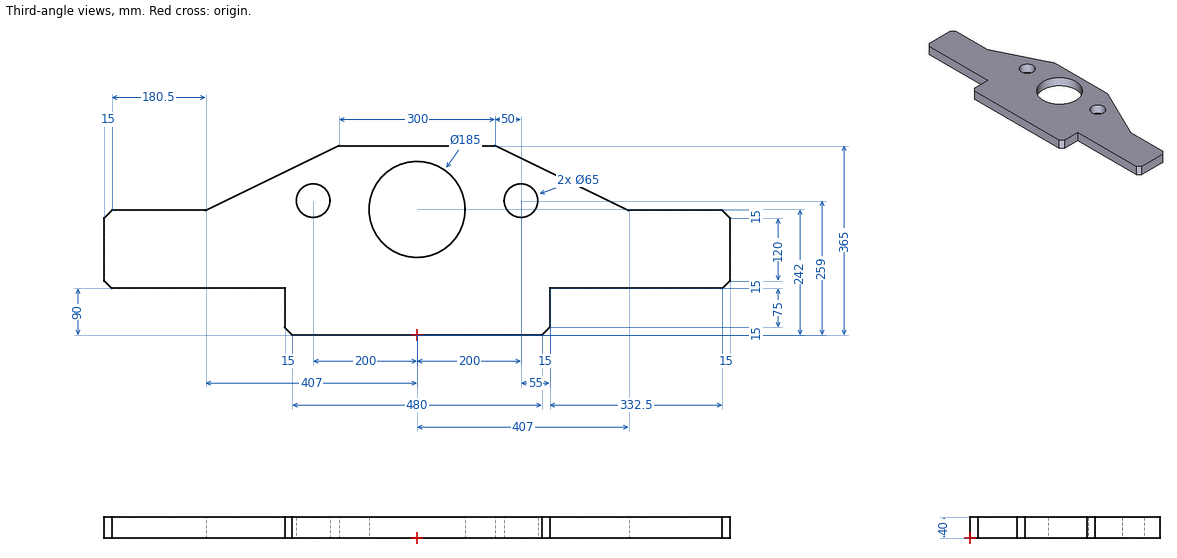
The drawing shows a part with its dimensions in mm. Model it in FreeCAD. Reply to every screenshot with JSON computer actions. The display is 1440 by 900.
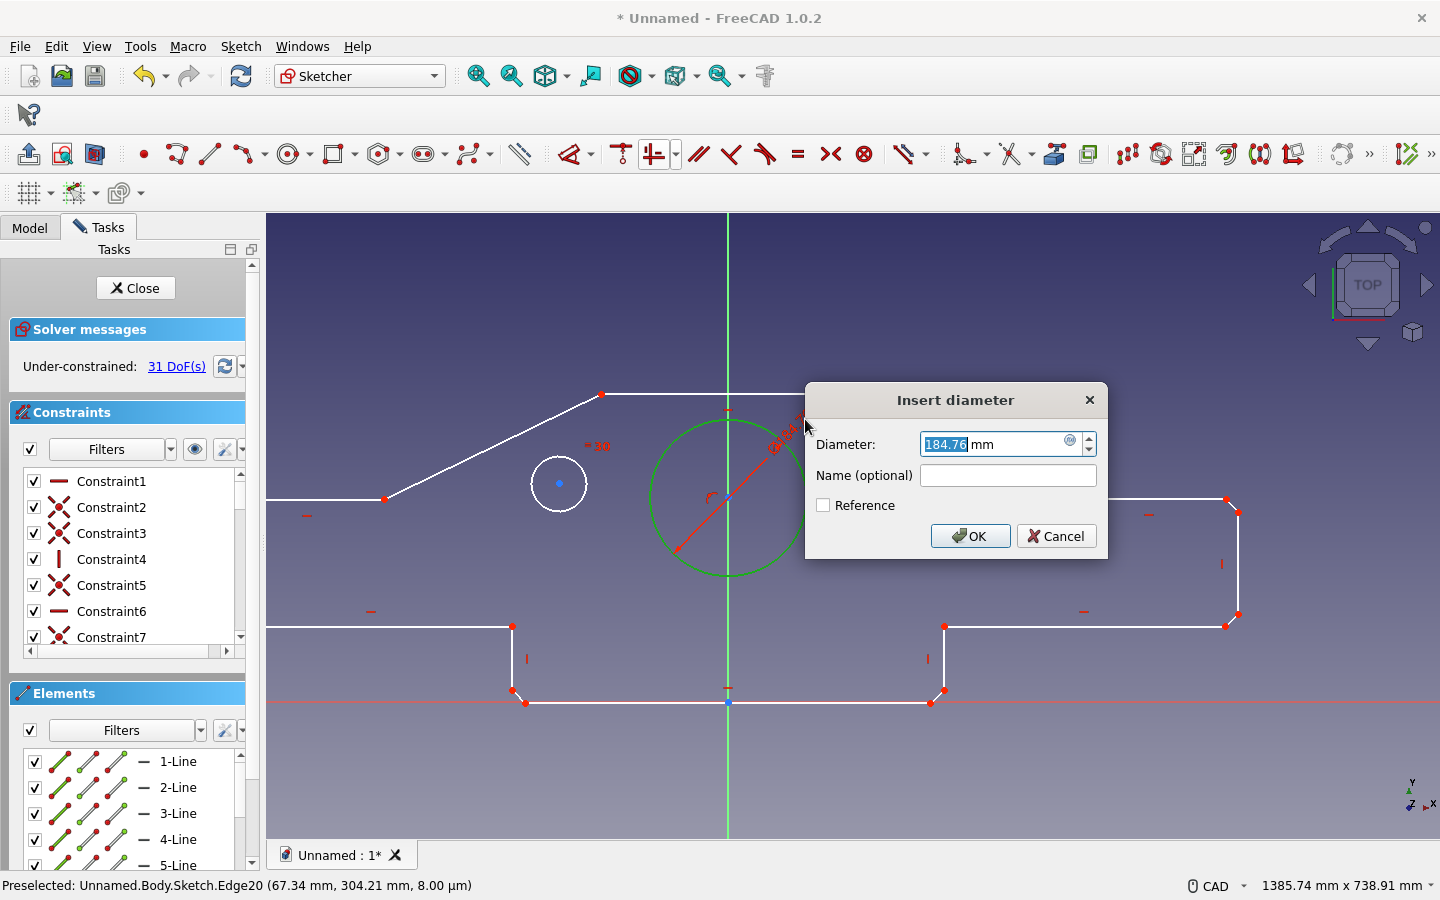
{"action": "type", "text": "185"}
{"action": "key", "text": "Return"}
{"action": "key", "text": "Escape"}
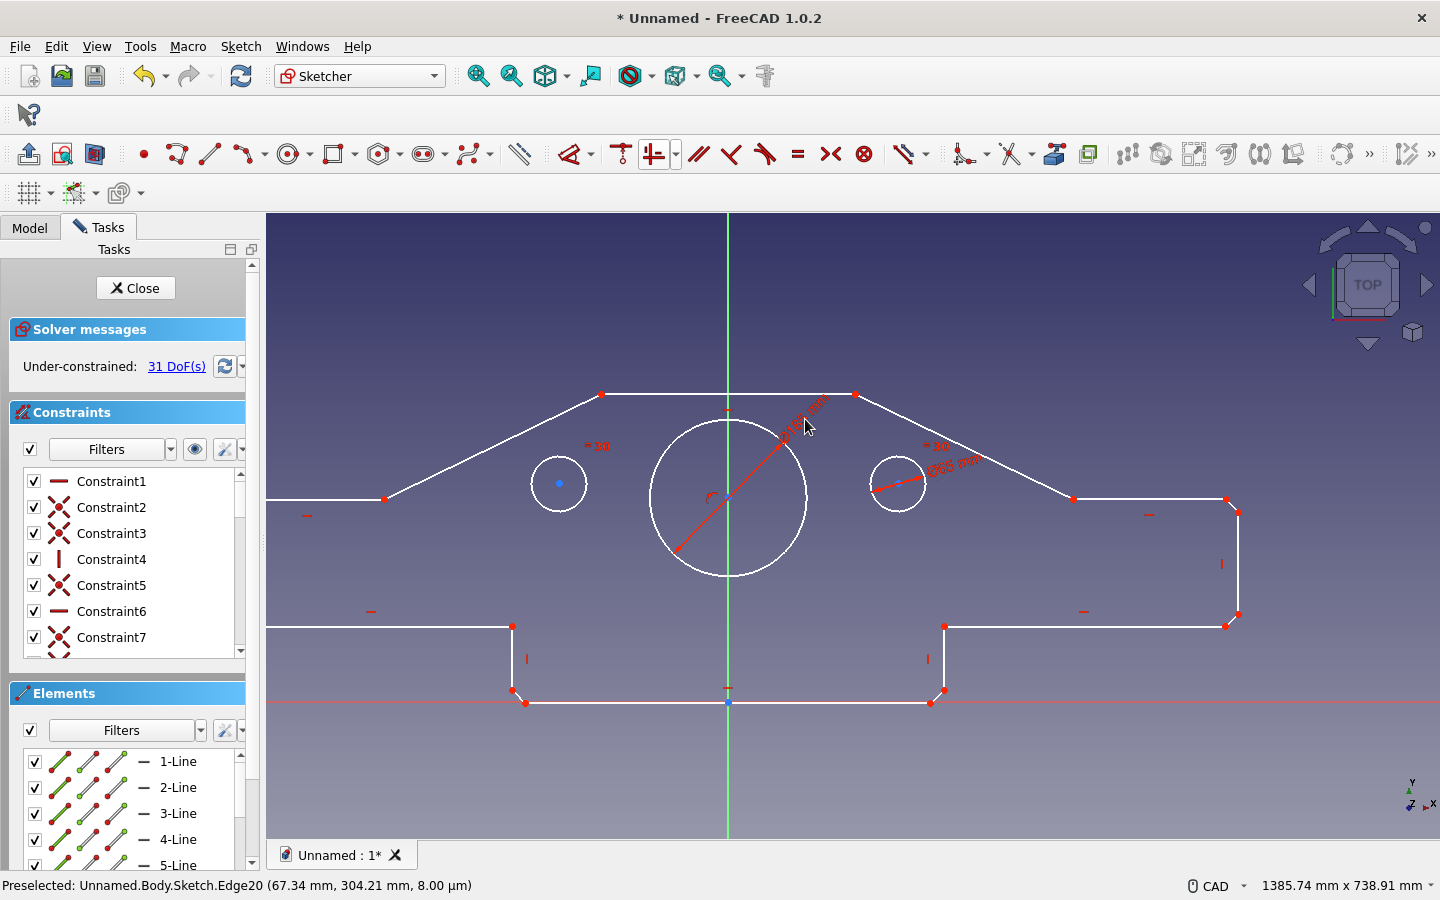
{"action": "left_click", "coordinate": [525, 703]}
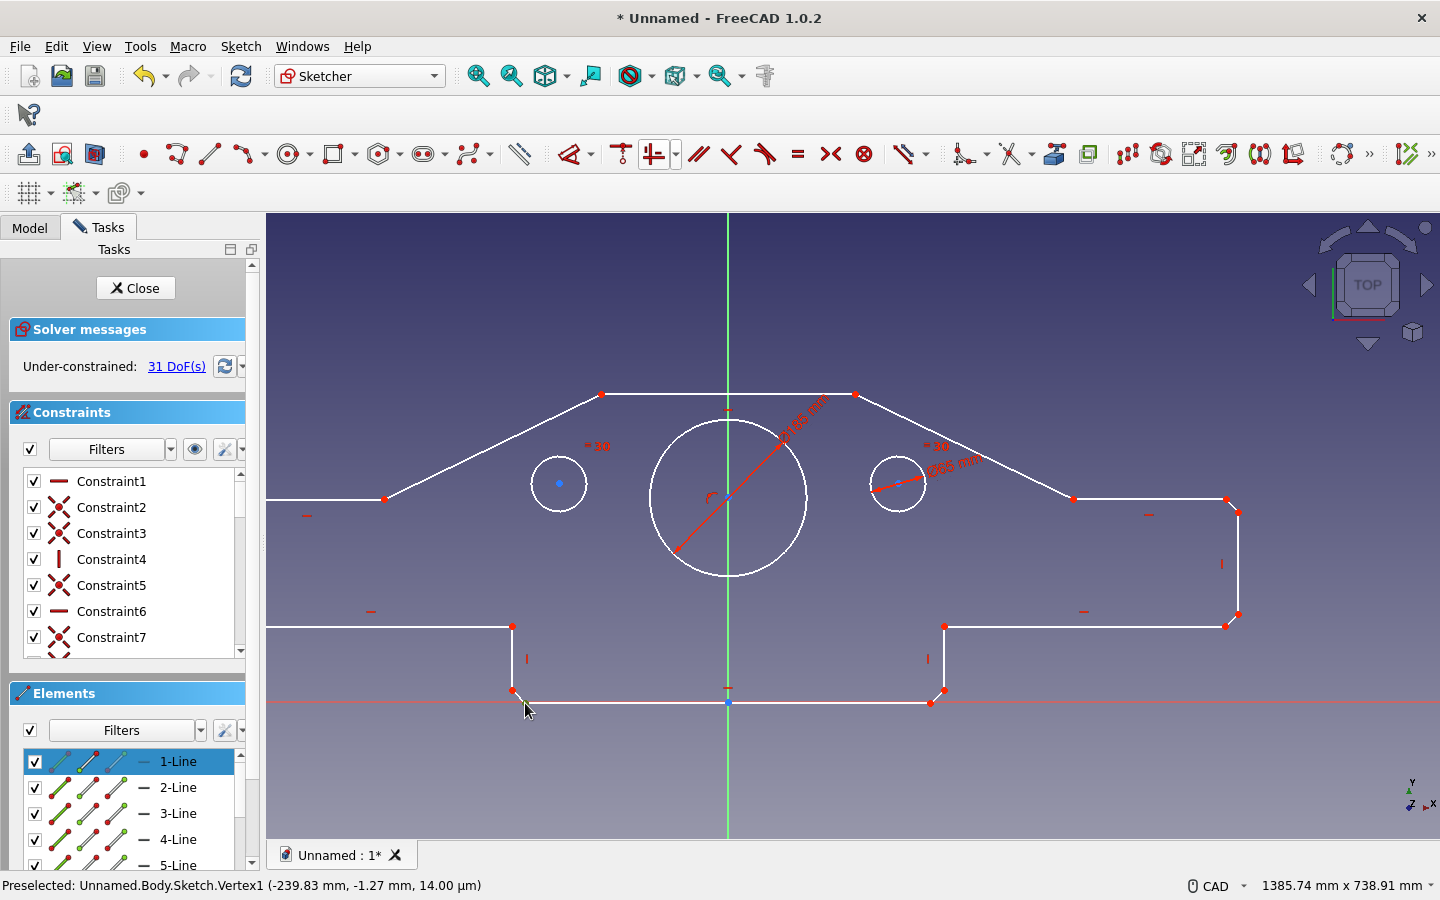
{"action": "left_click", "coordinate": [364, 702]}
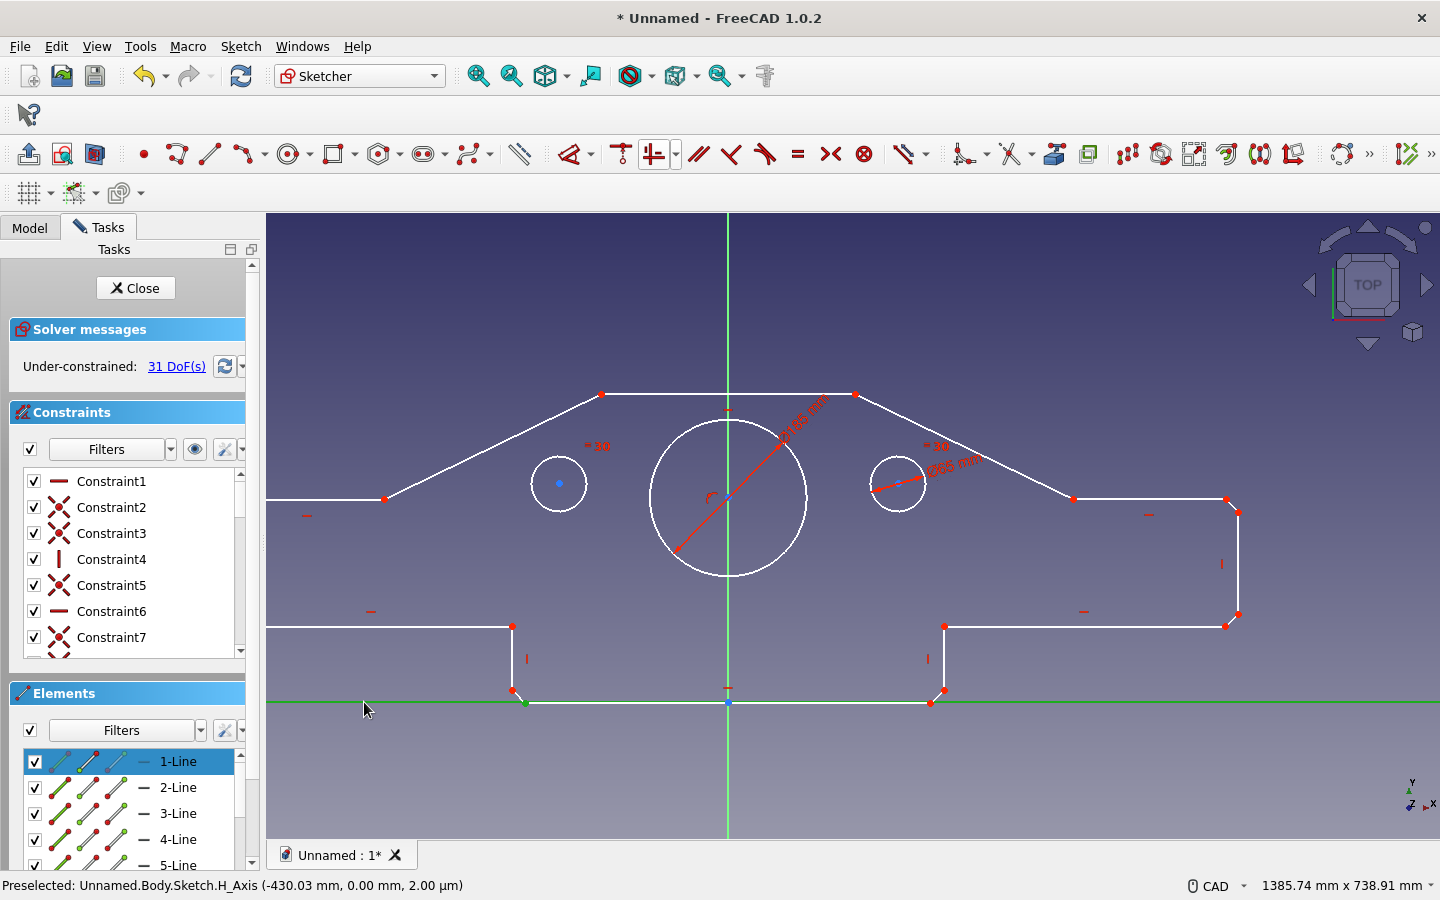
{"action": "left_click", "coordinate": [621, 154]}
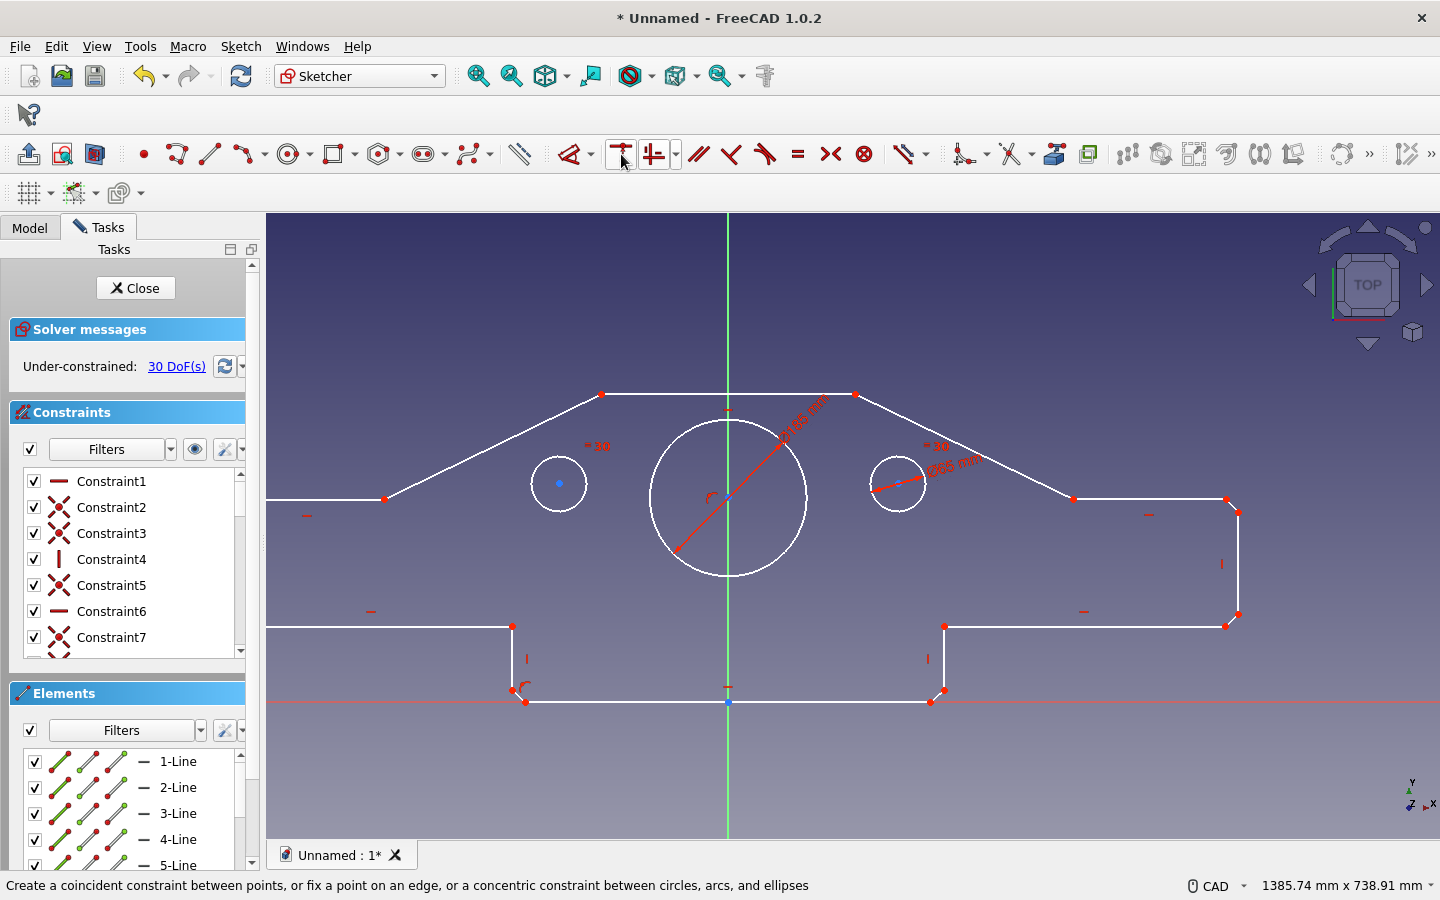
{"action": "left_click", "coordinate": [568, 154]}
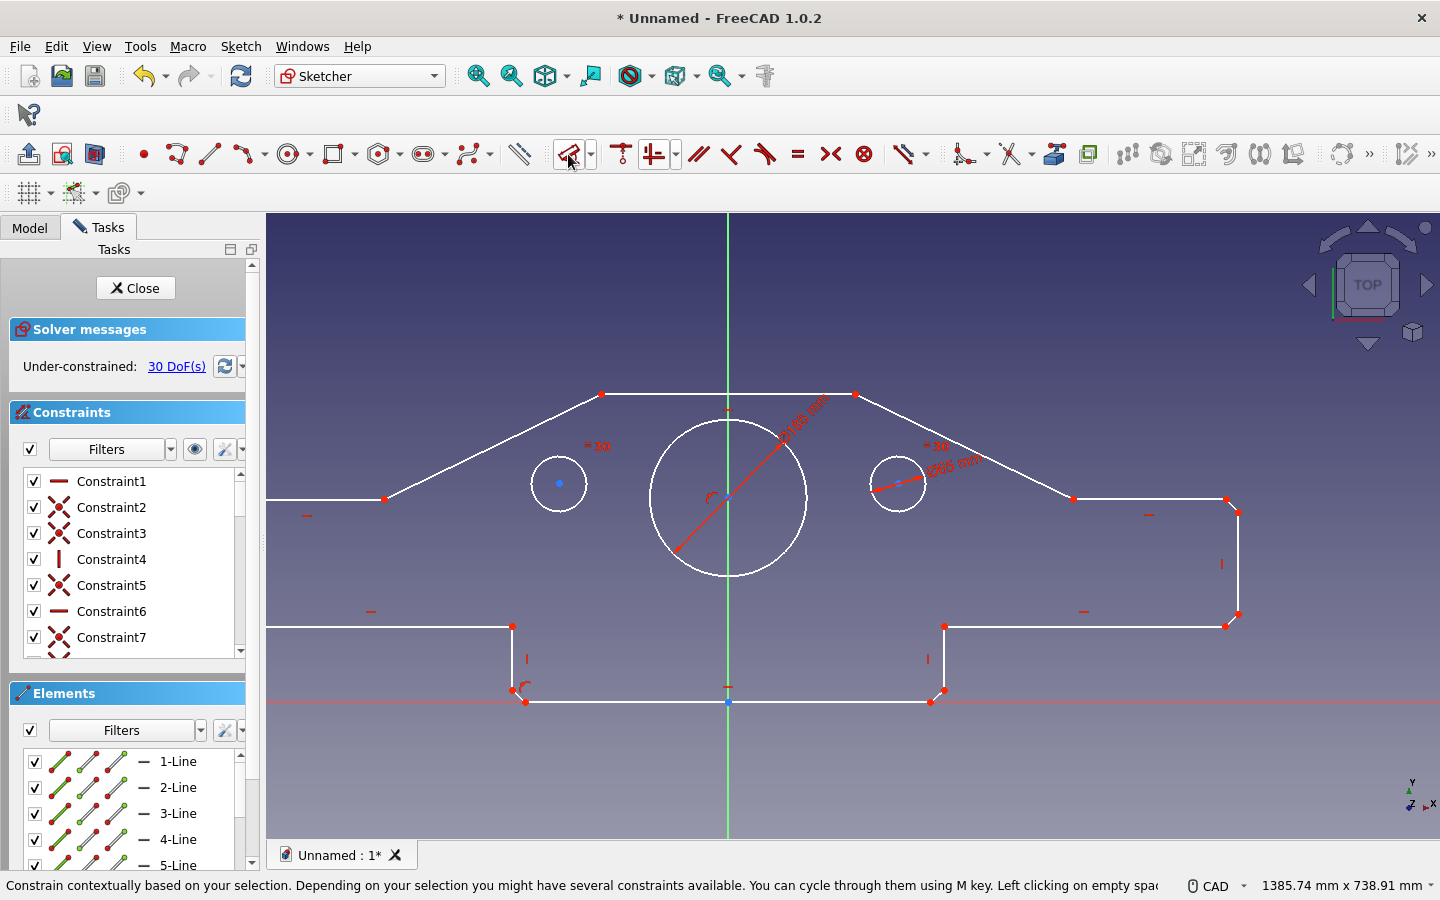
{"action": "left_click", "coordinate": [944, 671]}
{"action": "left_click", "coordinate": [978, 658]}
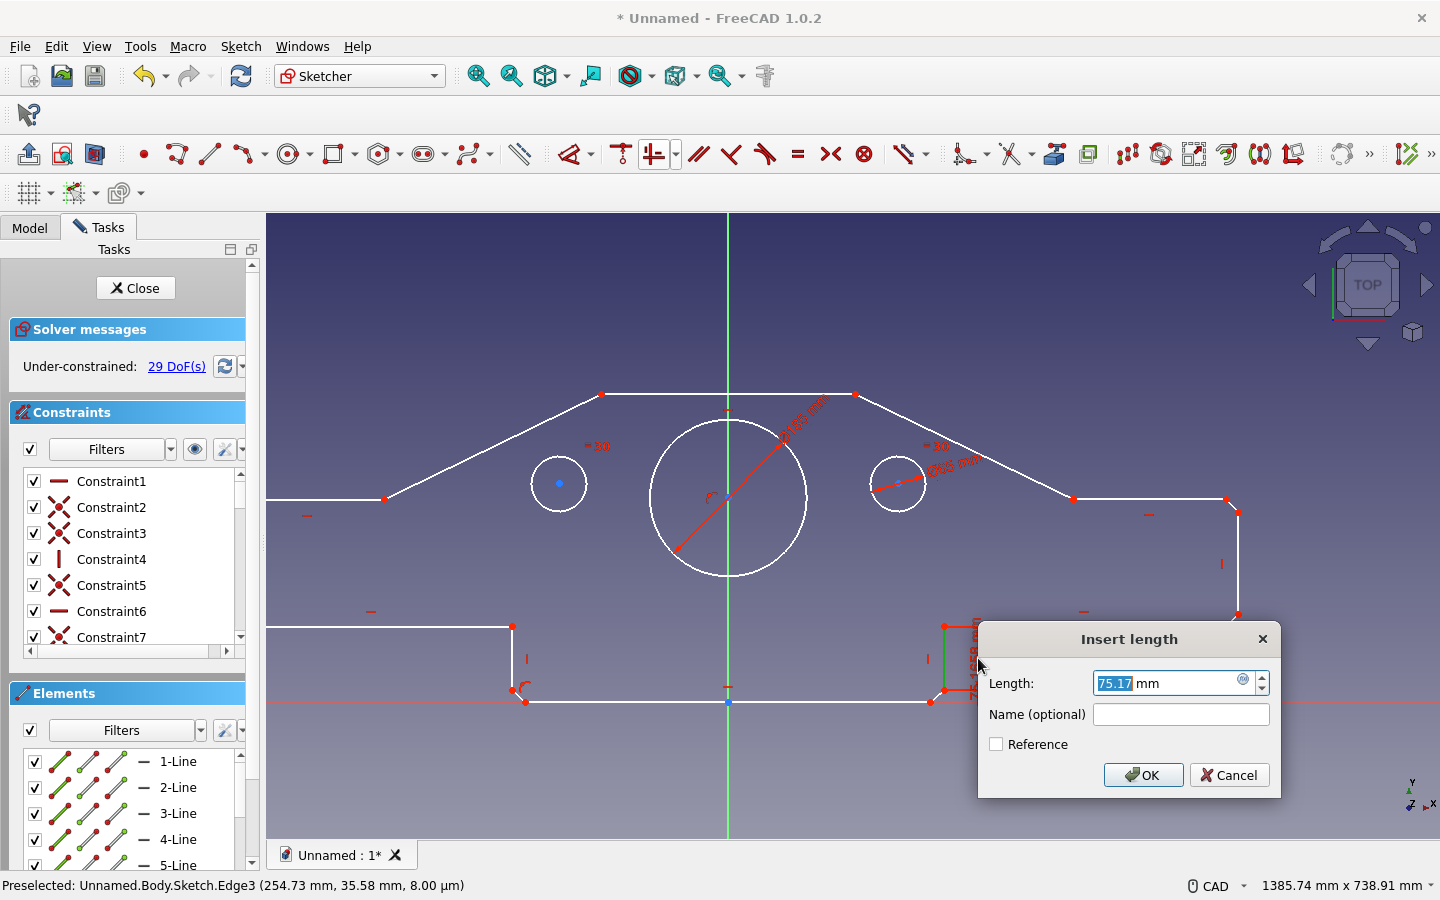
{"action": "type", "text": "75"}
{"action": "key", "text": "Return"}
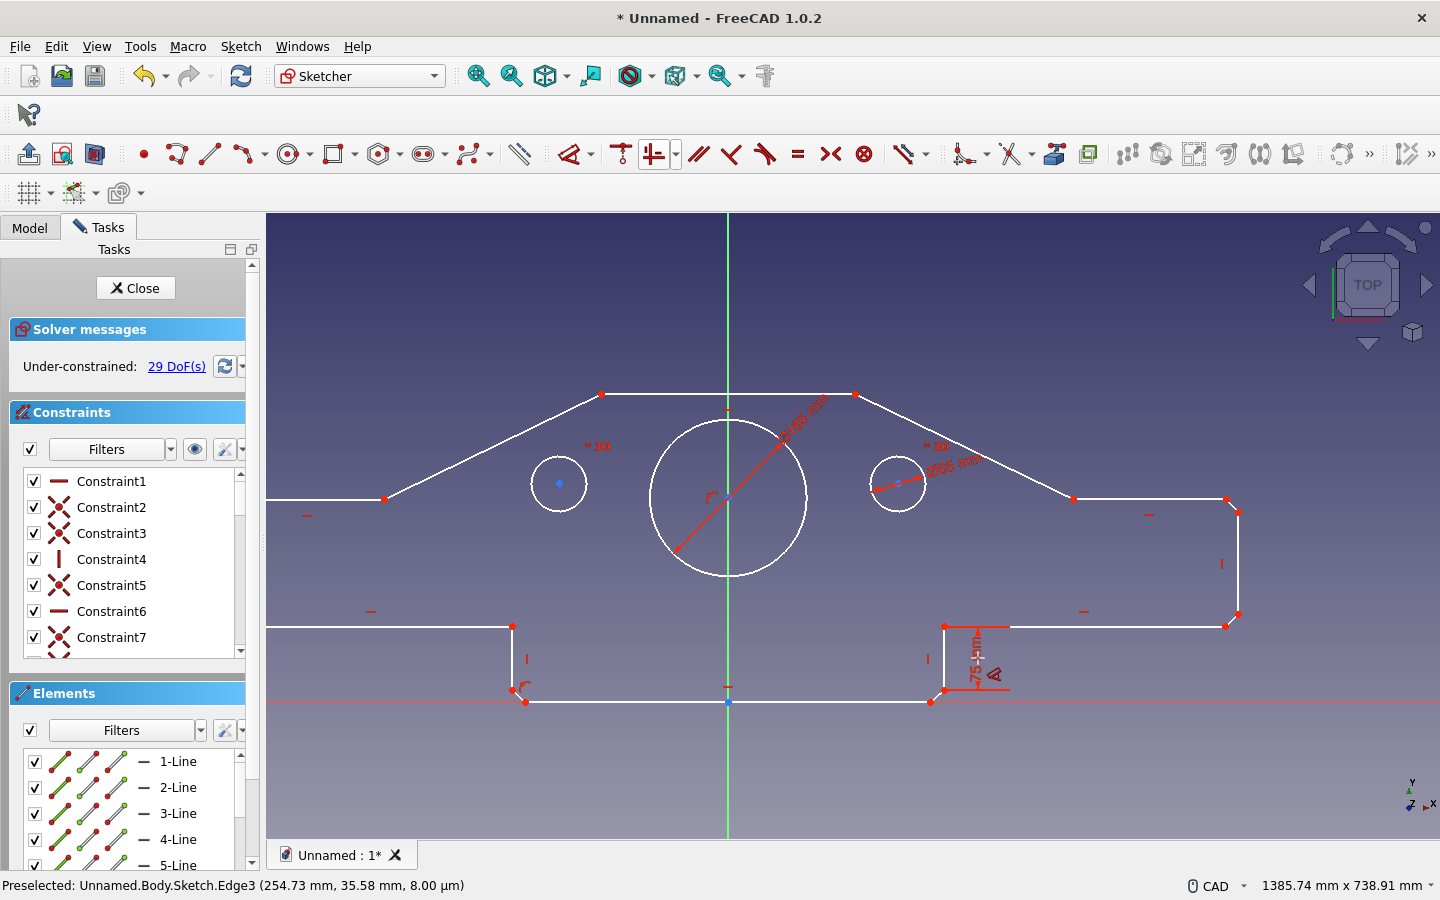
{"action": "left_click", "coordinate": [512, 646]}
{"action": "left_click", "coordinate": [478, 658]}